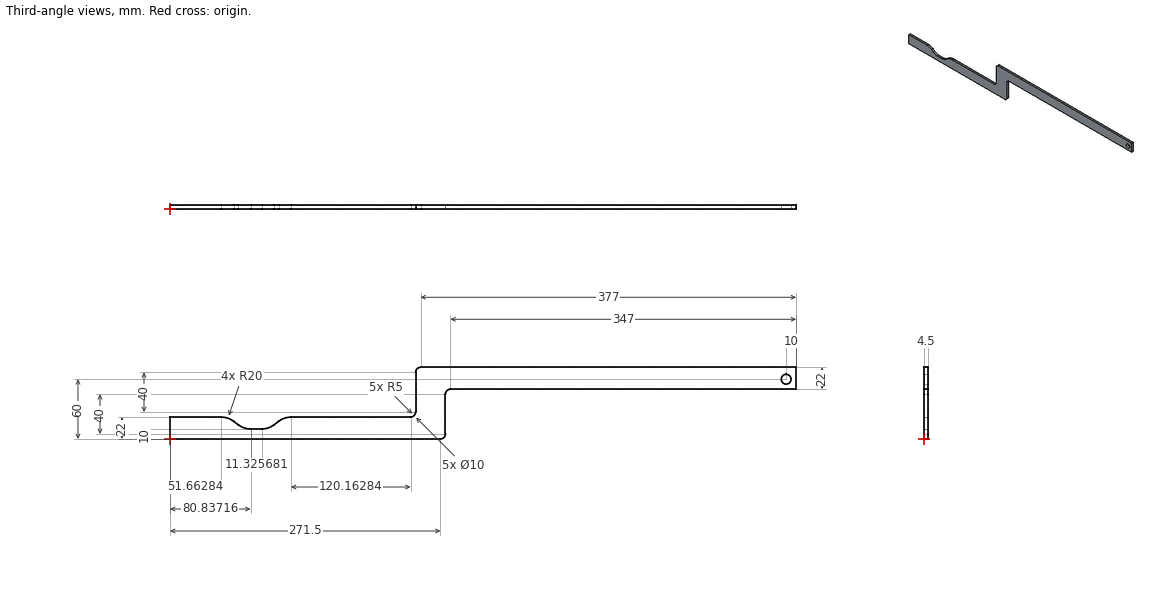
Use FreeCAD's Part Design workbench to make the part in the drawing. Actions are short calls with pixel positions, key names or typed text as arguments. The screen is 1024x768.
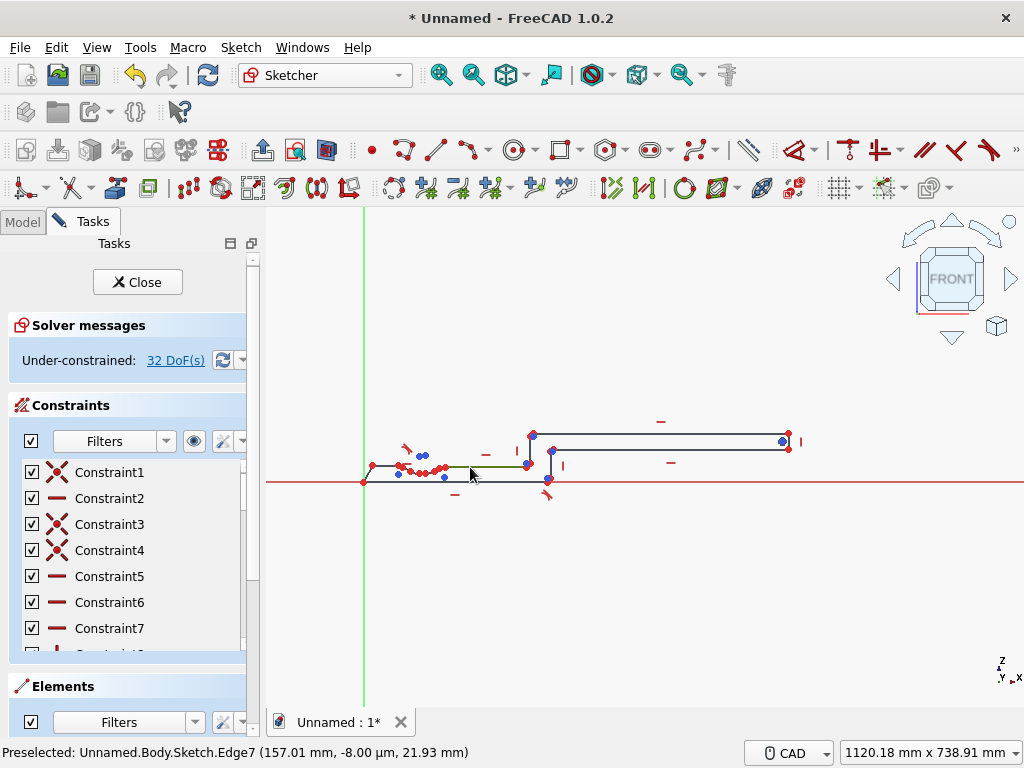
scroll(442, 467, up, 7)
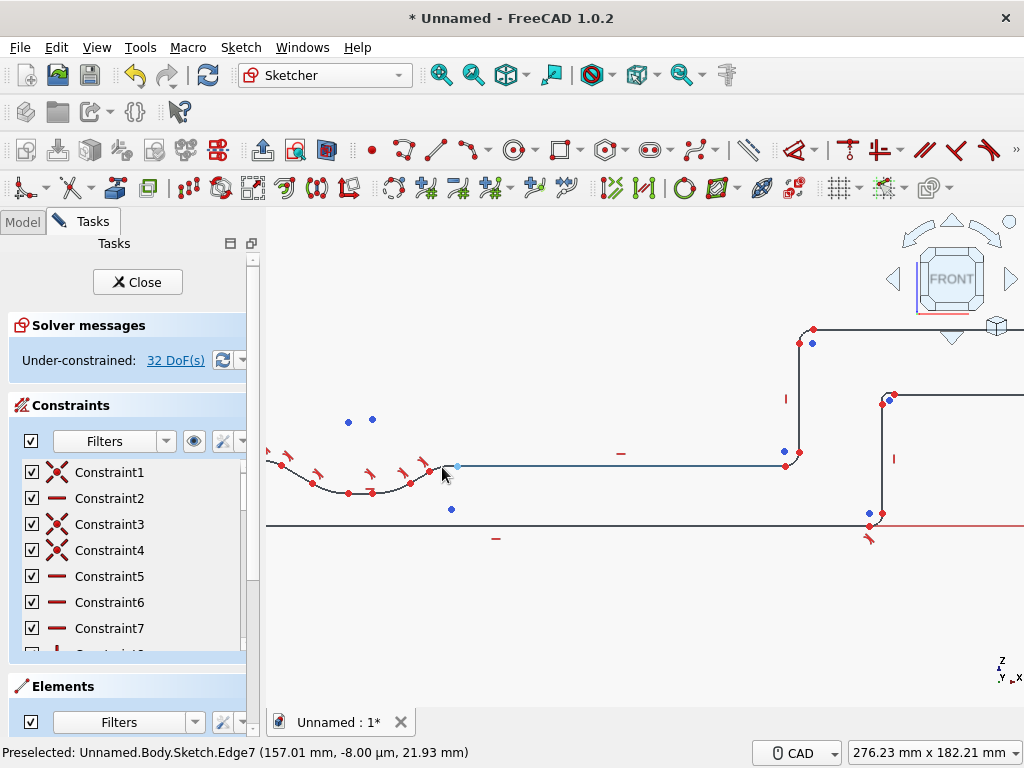
click(443, 467)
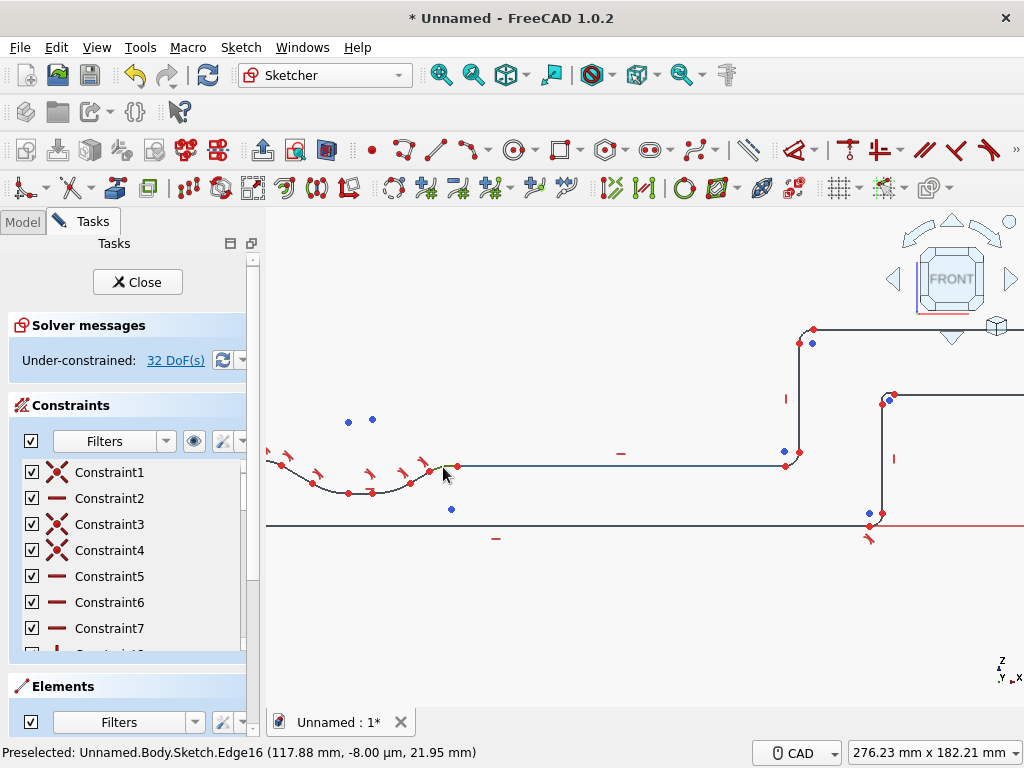
click(990, 150)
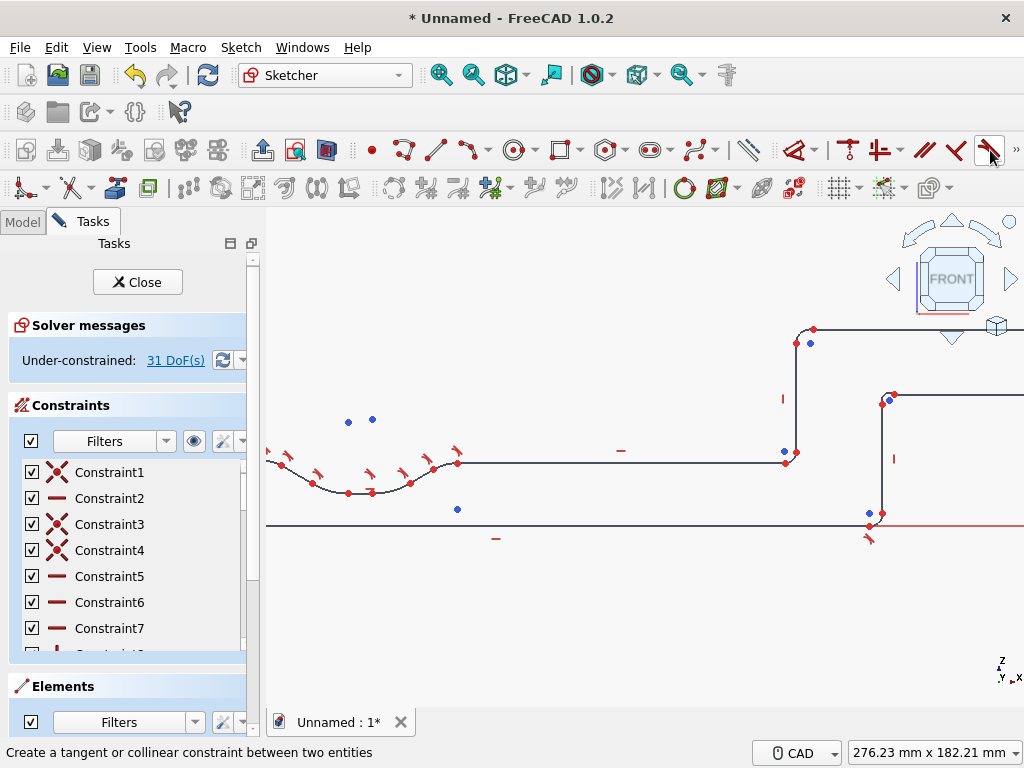
scroll(442, 467, down, 7)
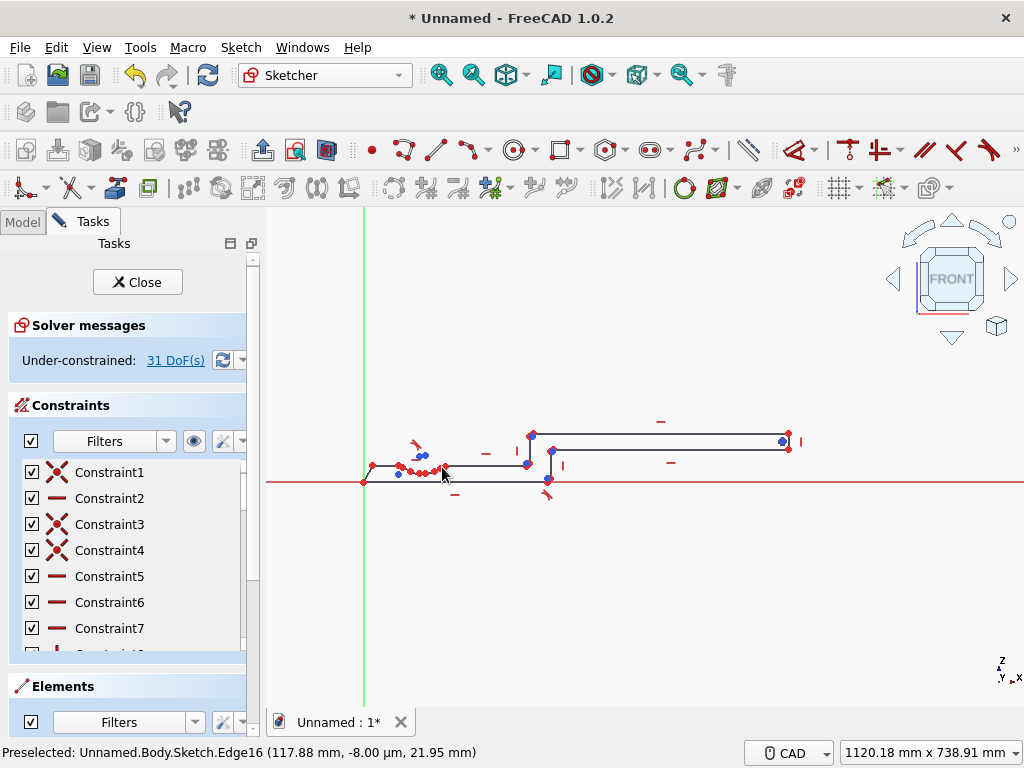
click(503, 466)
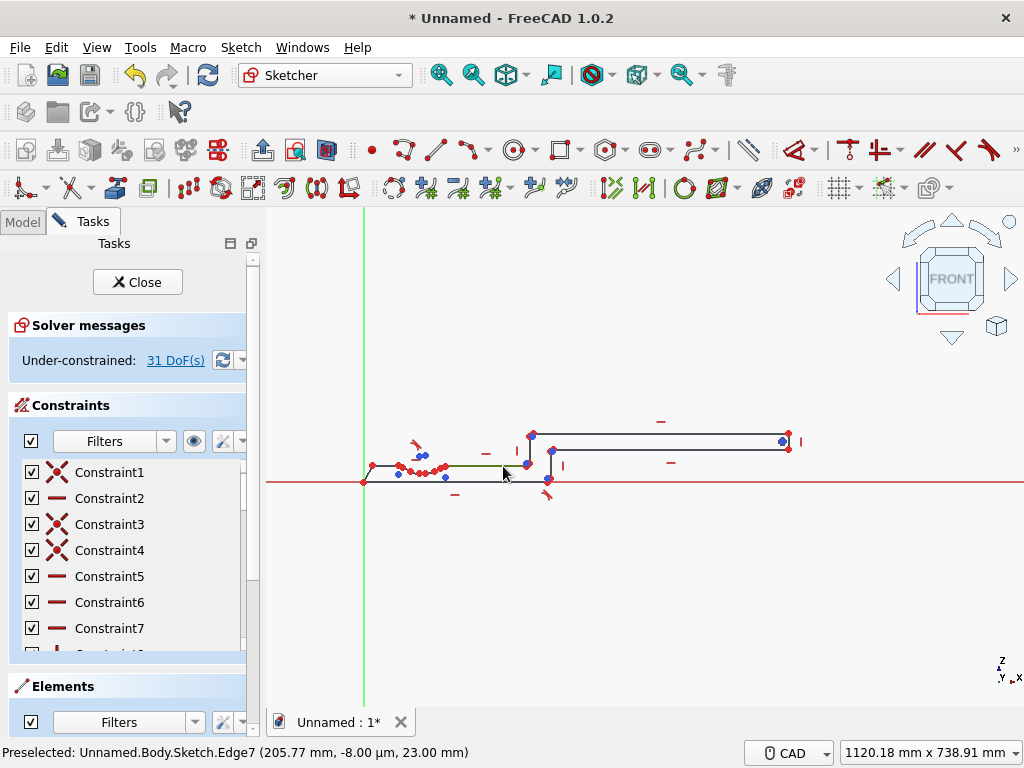
scroll(529, 466, up, 10)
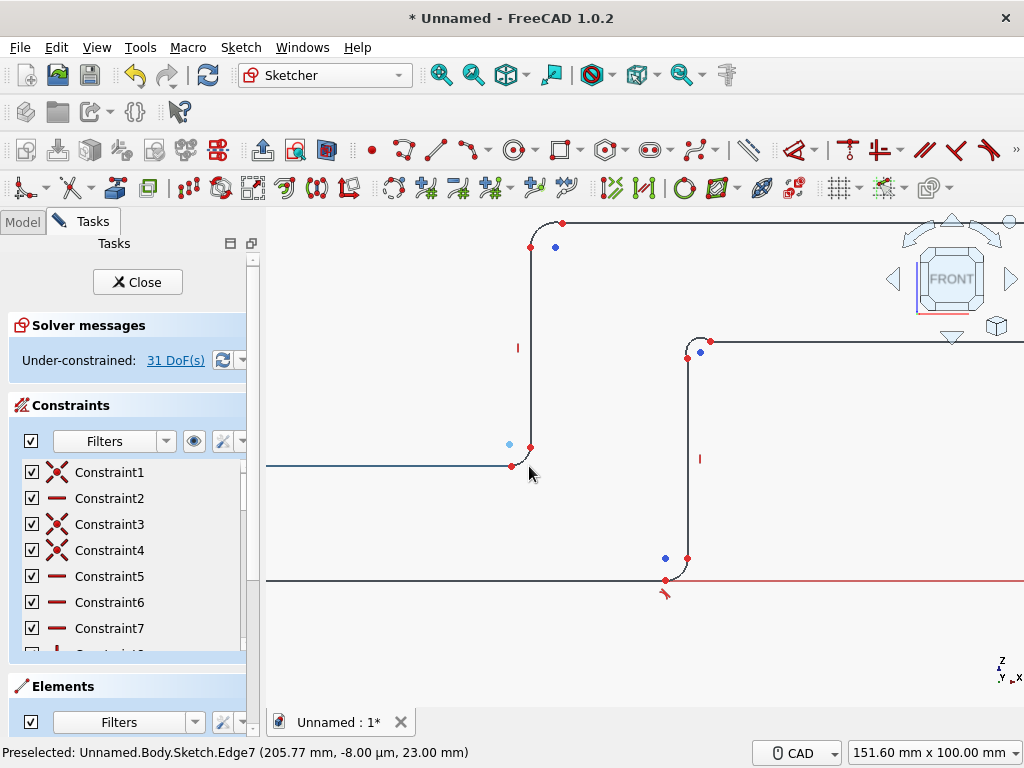
click(524, 460)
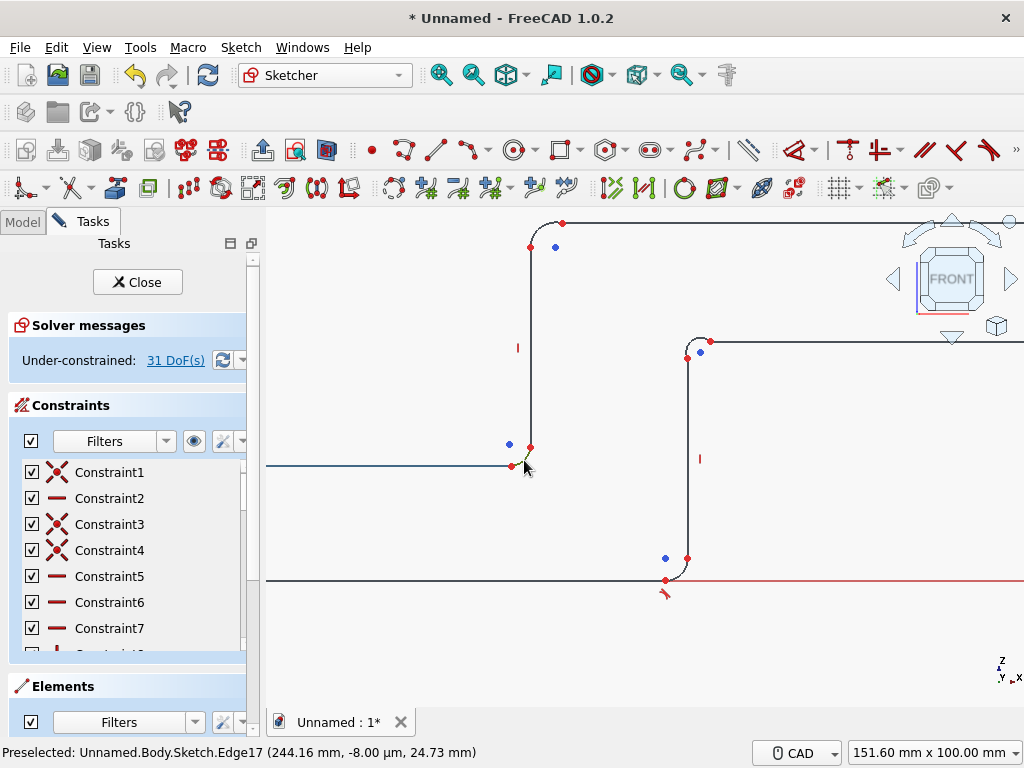
key(t)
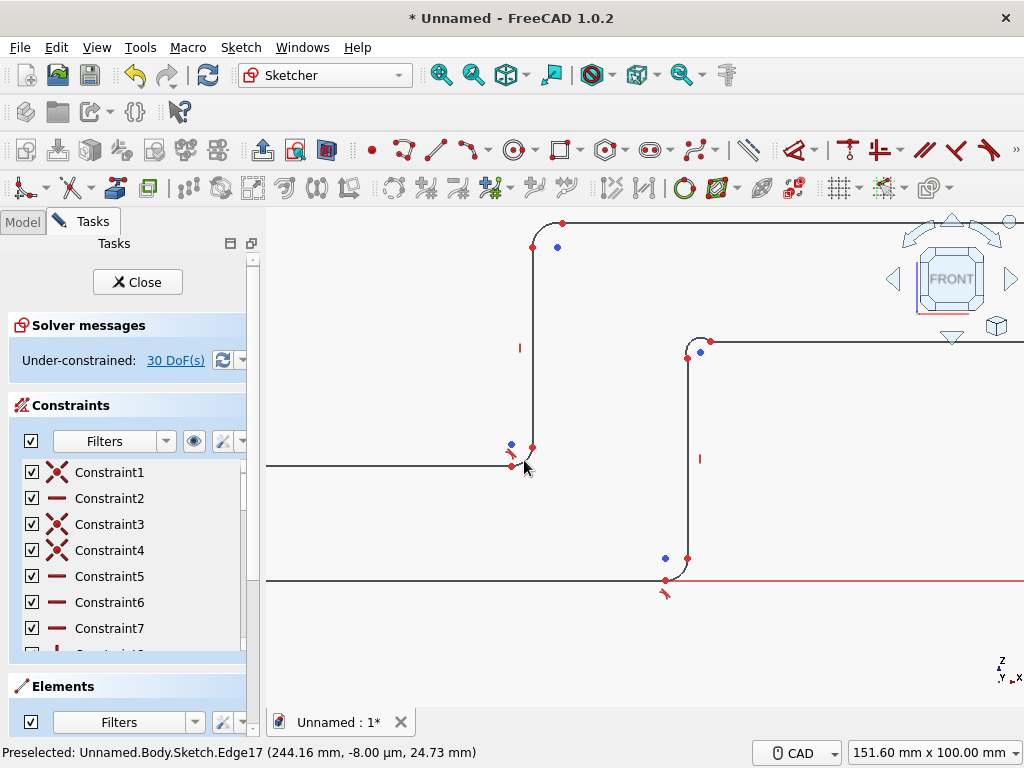
scroll(529, 466, down, 10)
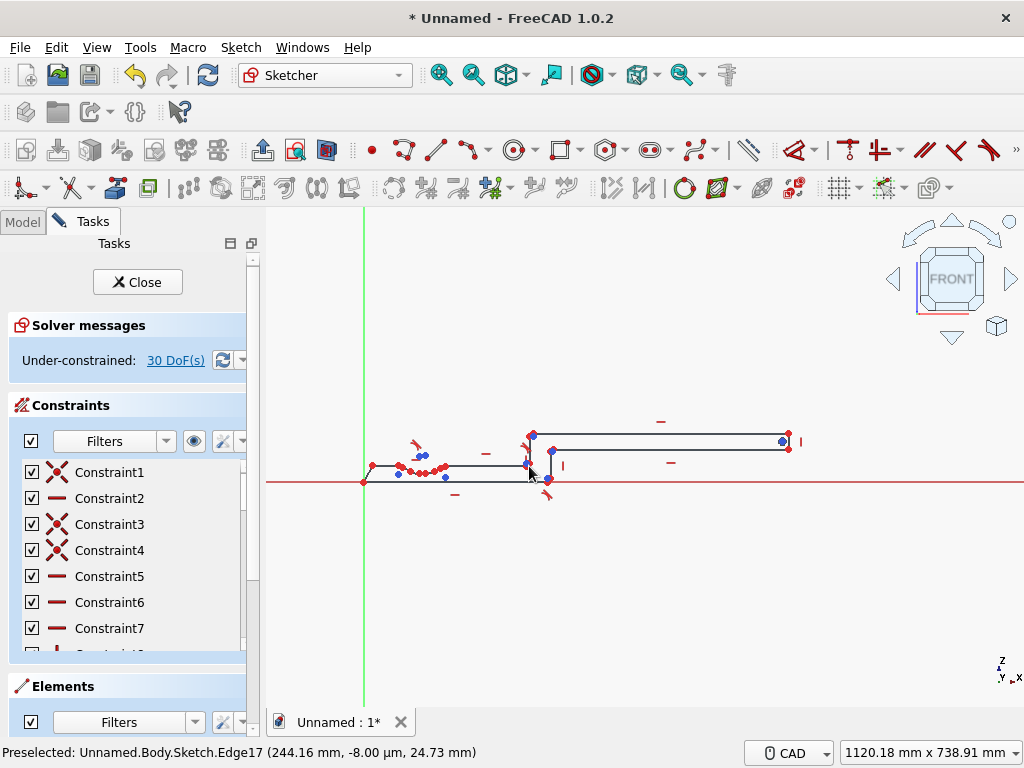
scroll(530, 456, up, 3)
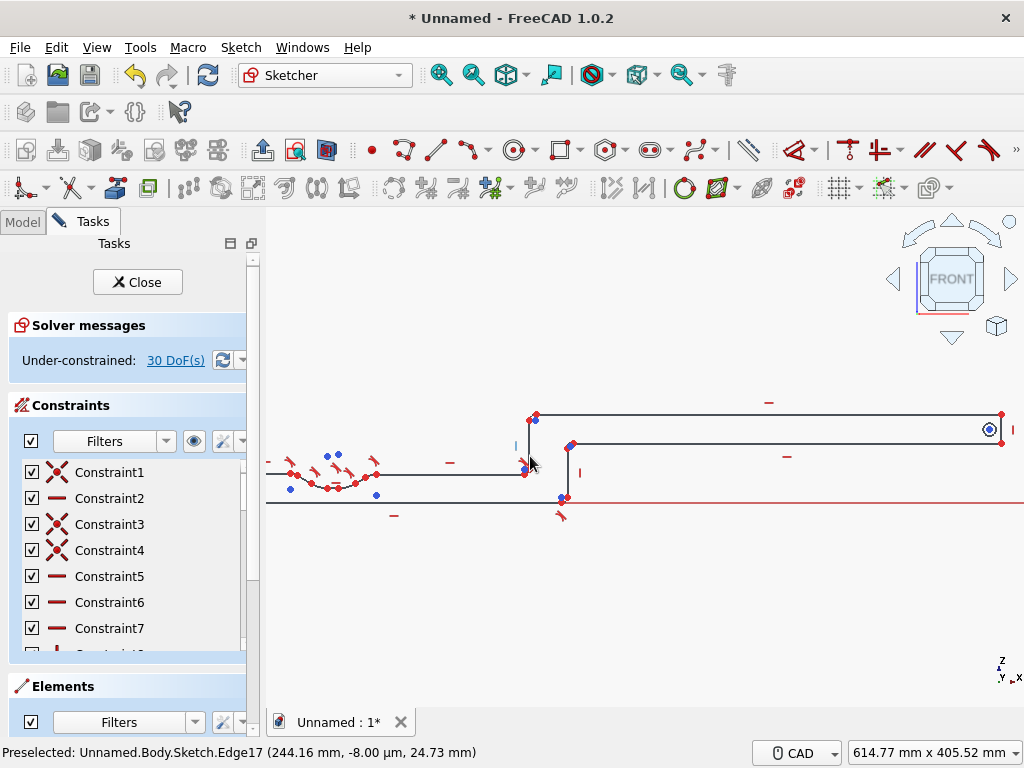
click(529, 455)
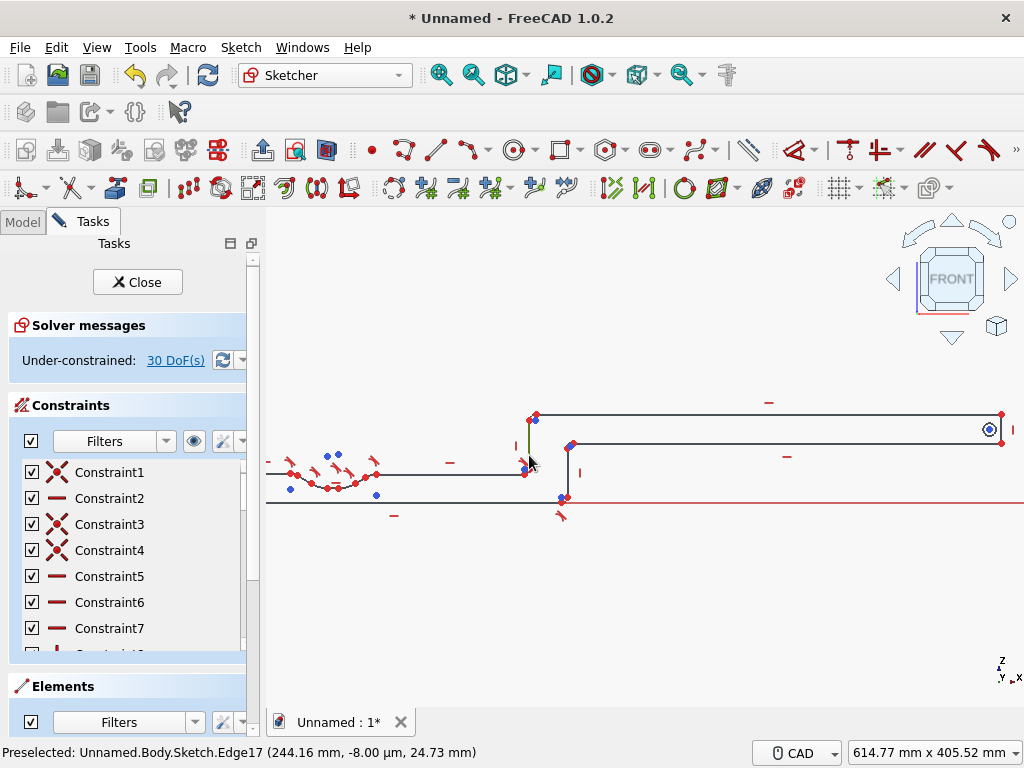
scroll(528, 473, up, 7)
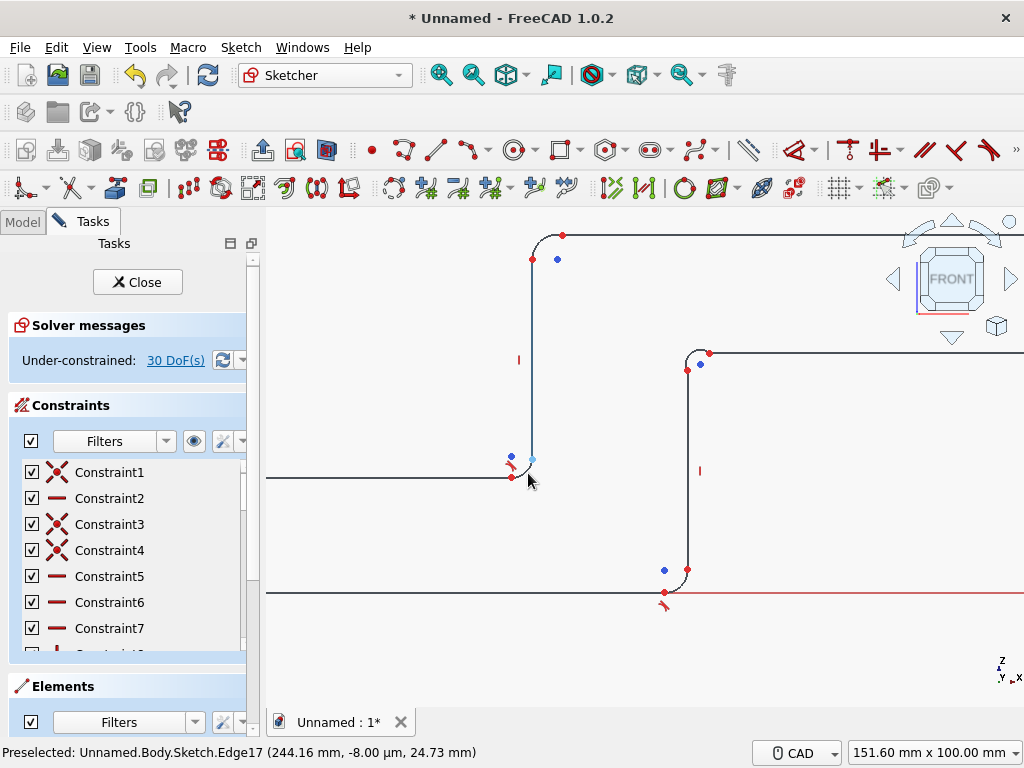
click(525, 473)